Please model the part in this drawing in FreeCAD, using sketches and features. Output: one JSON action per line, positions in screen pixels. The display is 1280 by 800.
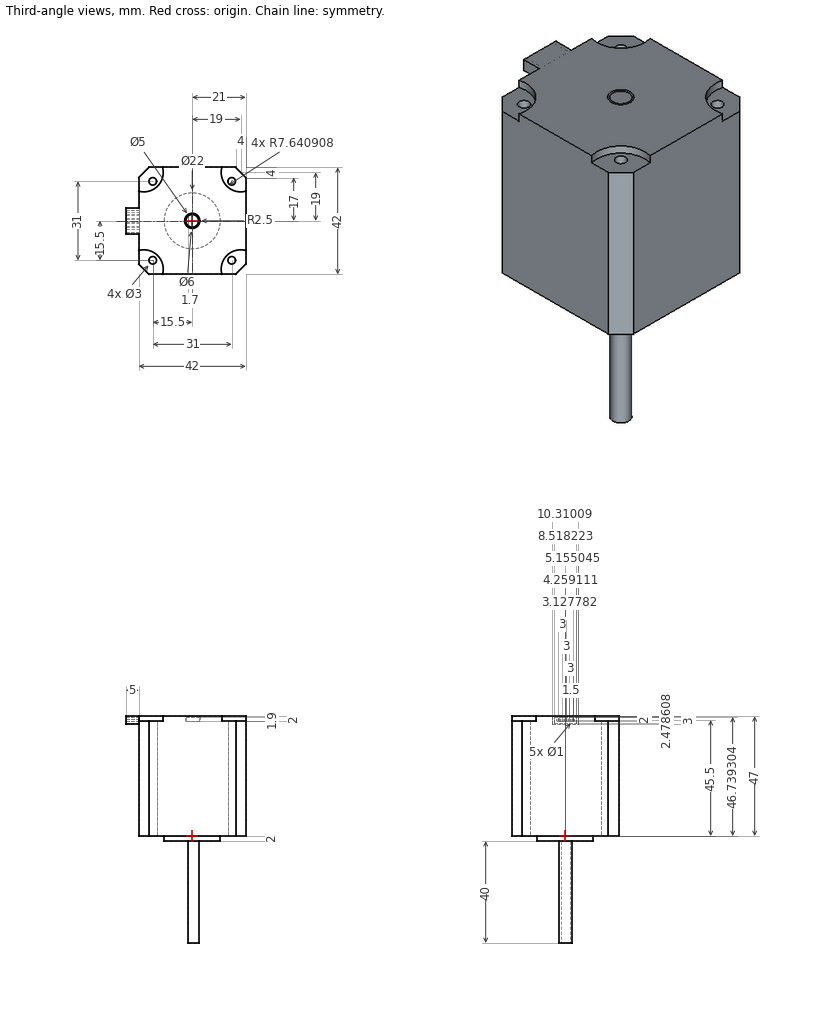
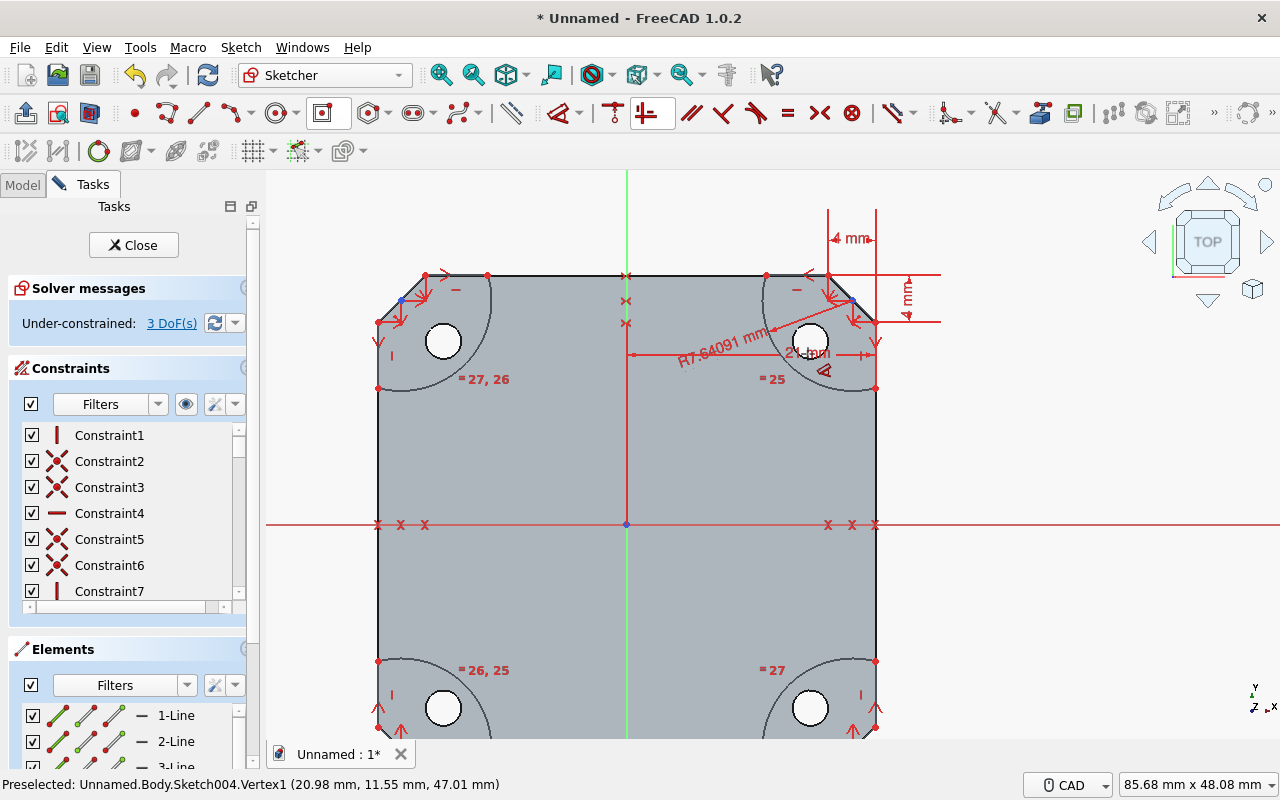
{"action": "left_click", "coordinate": [876, 322]}
{"action": "left_click", "coordinate": [910, 424]}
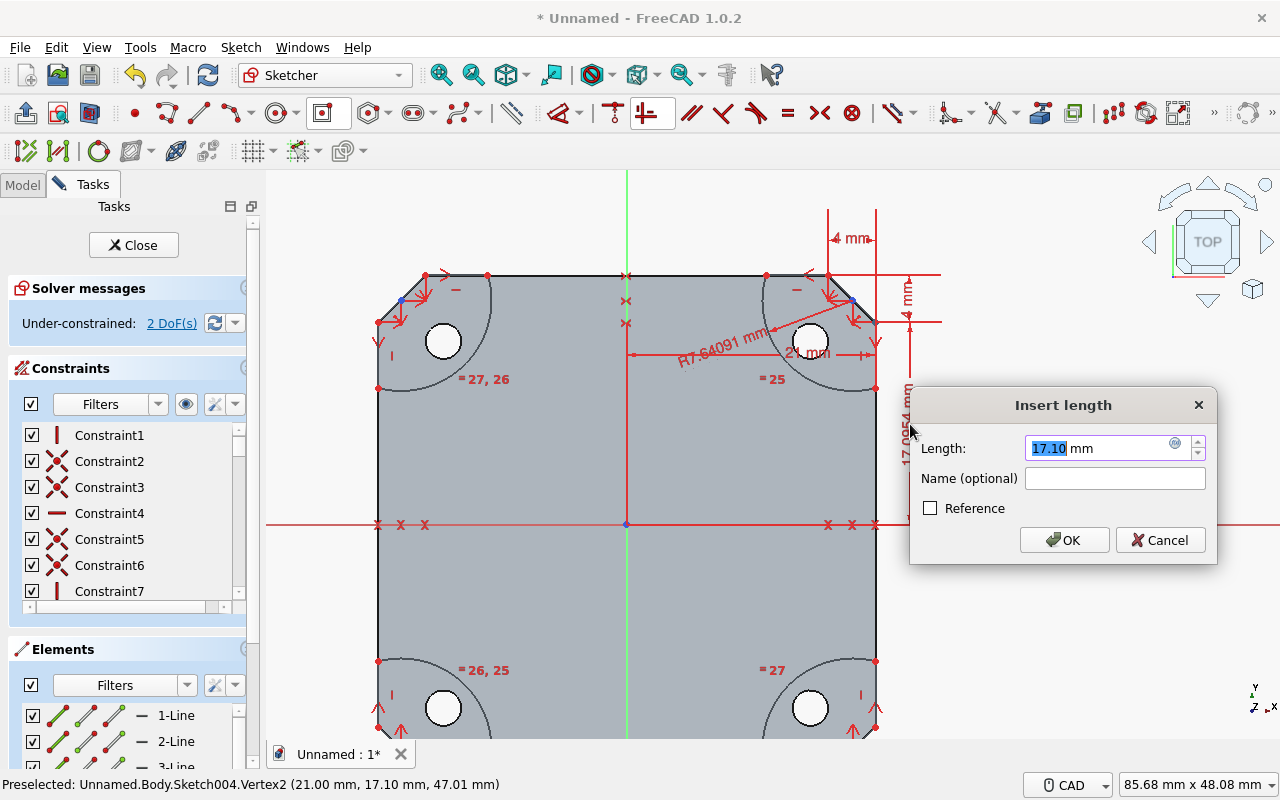
{"action": "type", "text": "17"}
{"action": "key", "text": "Return"}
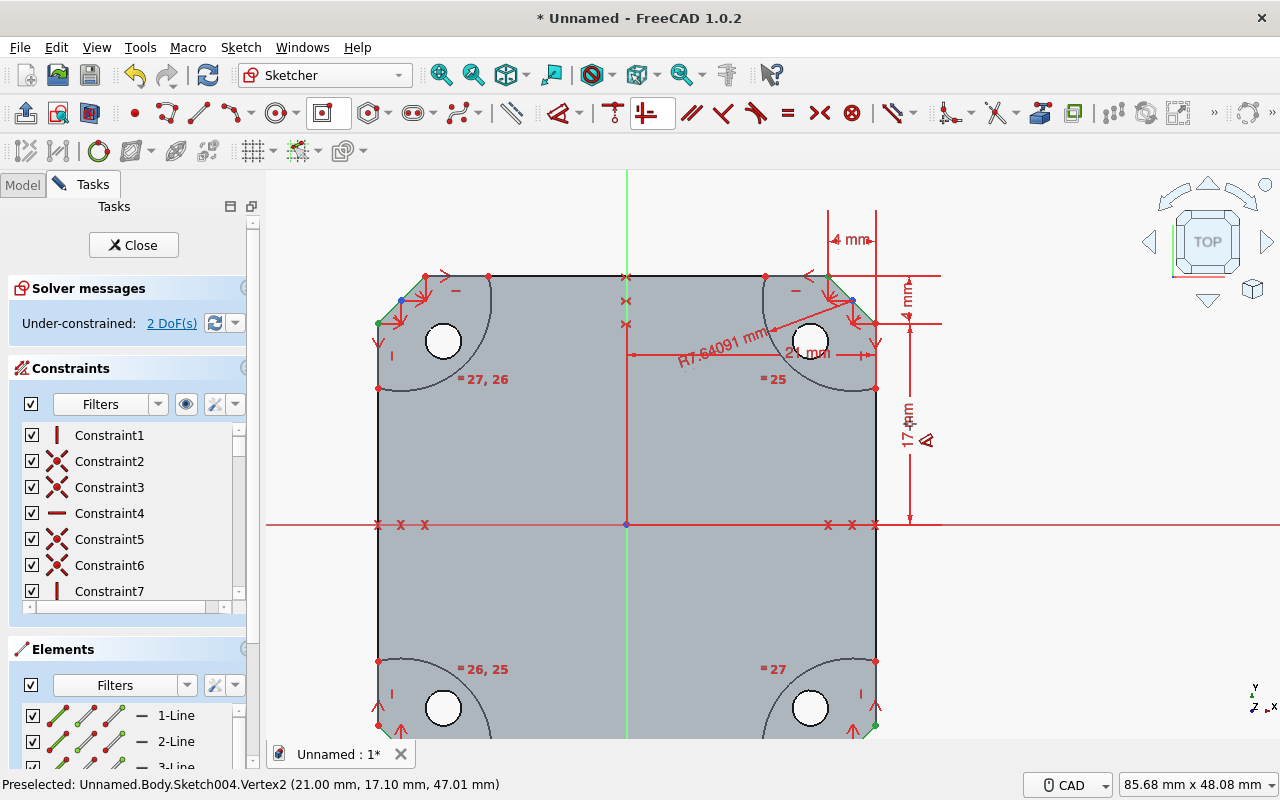
{"action": "left_click", "coordinate": [853, 301]}
{"action": "left_click", "coordinate": [740, 267]}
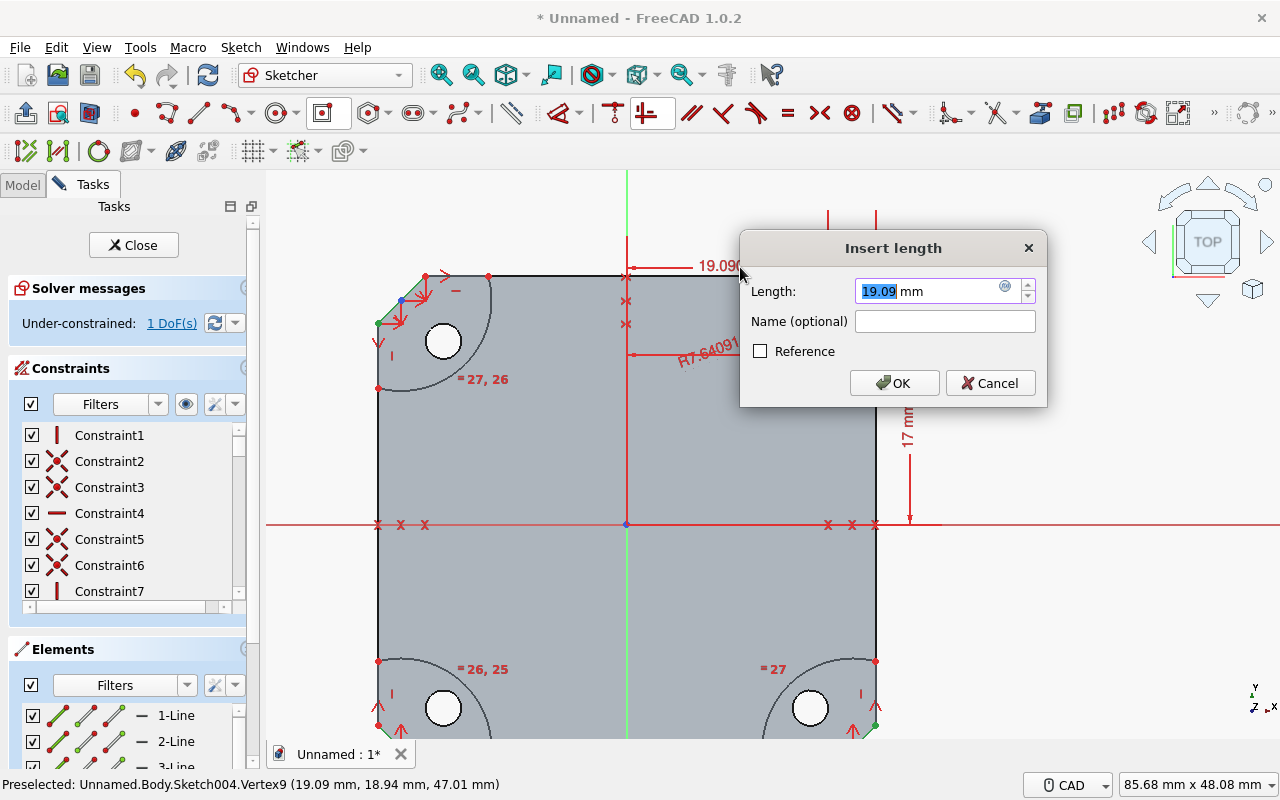
{"action": "type", "text": "19"}
{"action": "key", "text": "Return"}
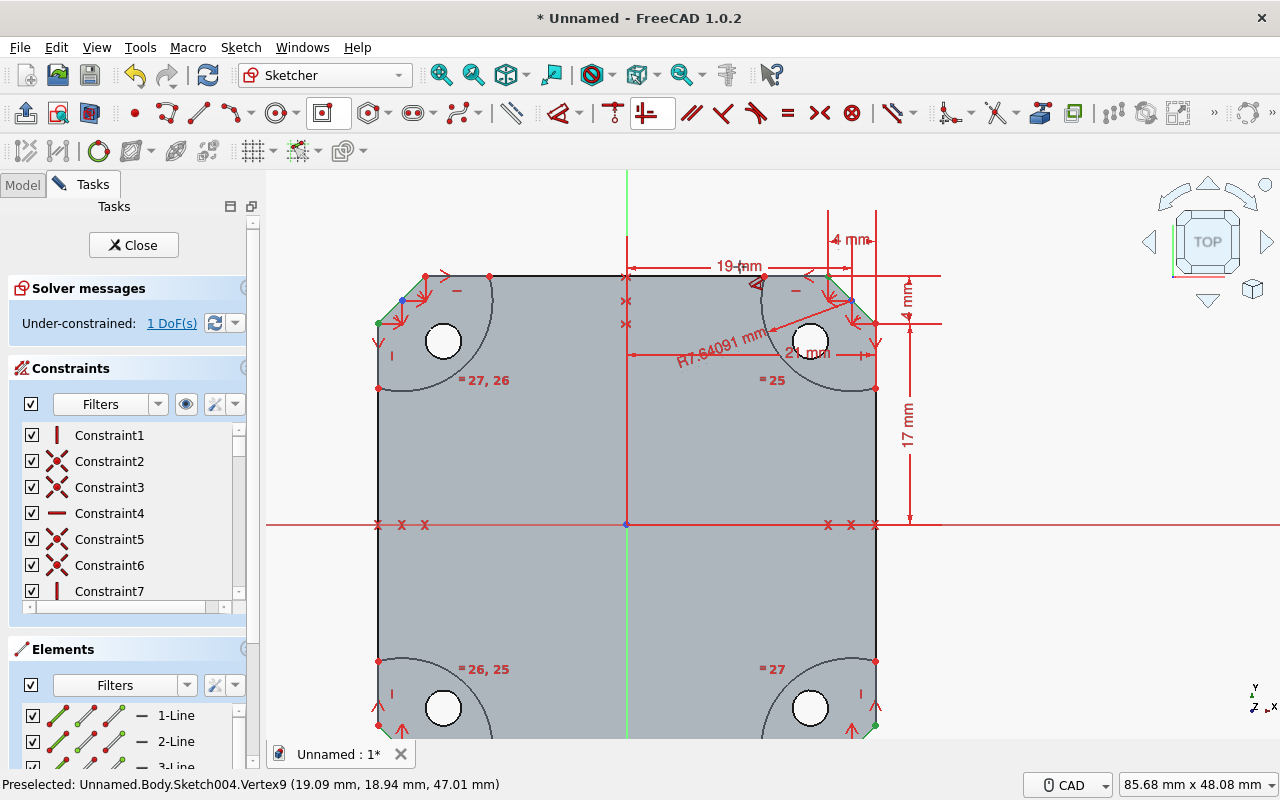
{"action": "left_click", "coordinate": [852, 301]}
{"action": "left_click", "coordinate": [886, 464]}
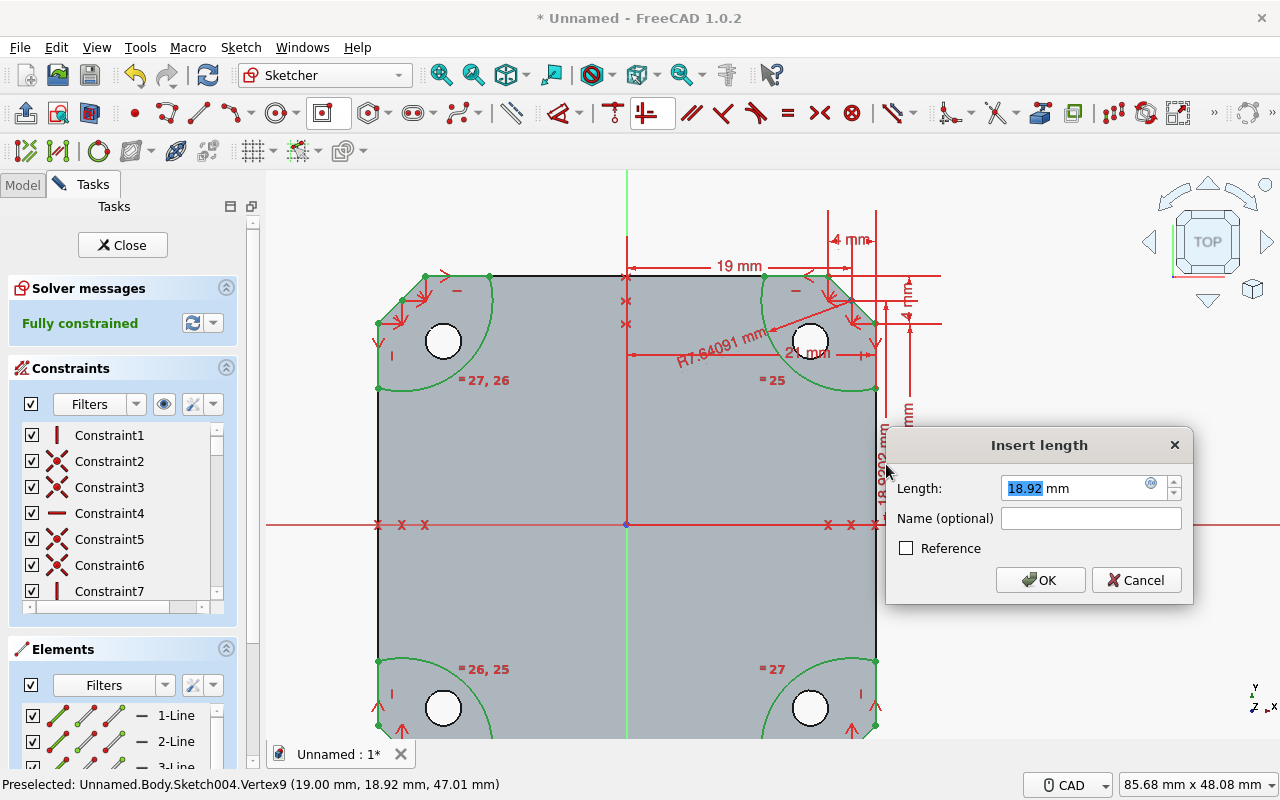
{"action": "type", "text": "19"}
{"action": "key", "text": "Return"}
{"action": "key", "text": "Escape"}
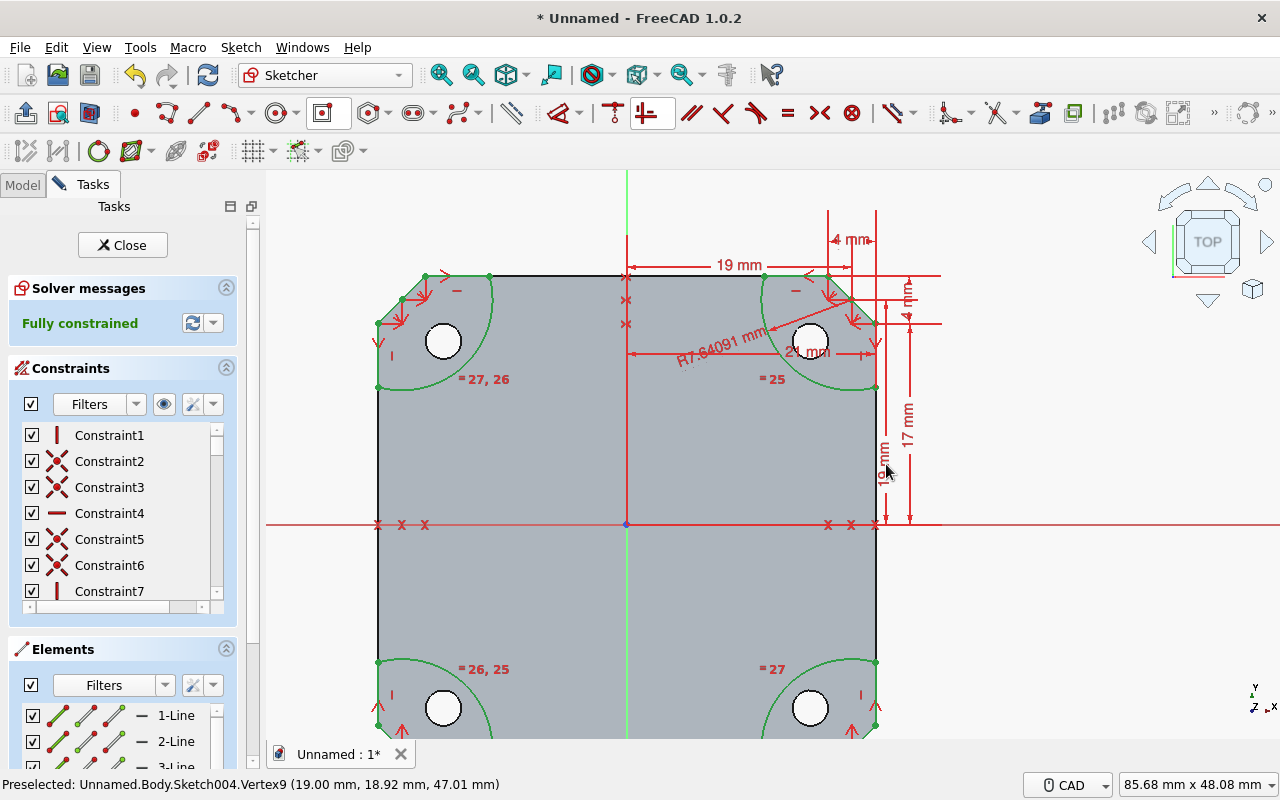
{"action": "left_click", "coordinate": [123, 245]}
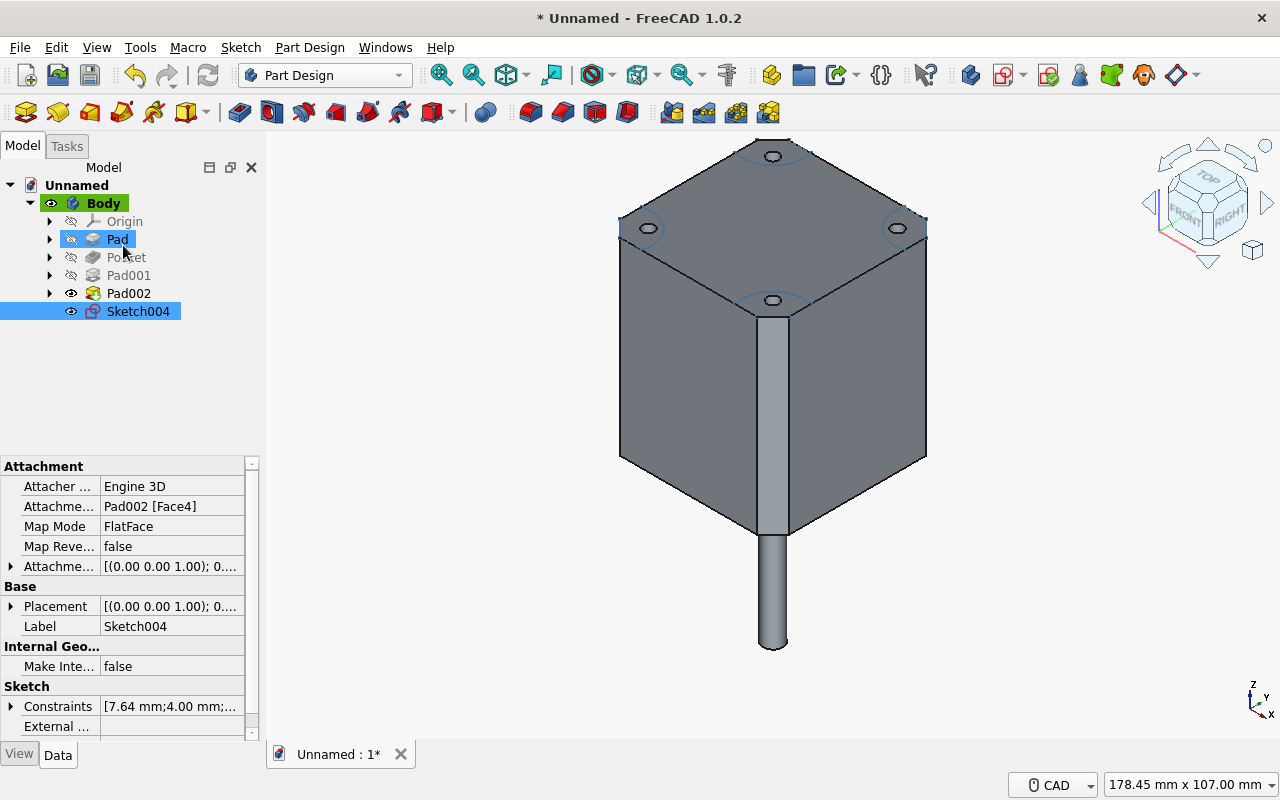
{"action": "left_click", "coordinate": [240, 112]}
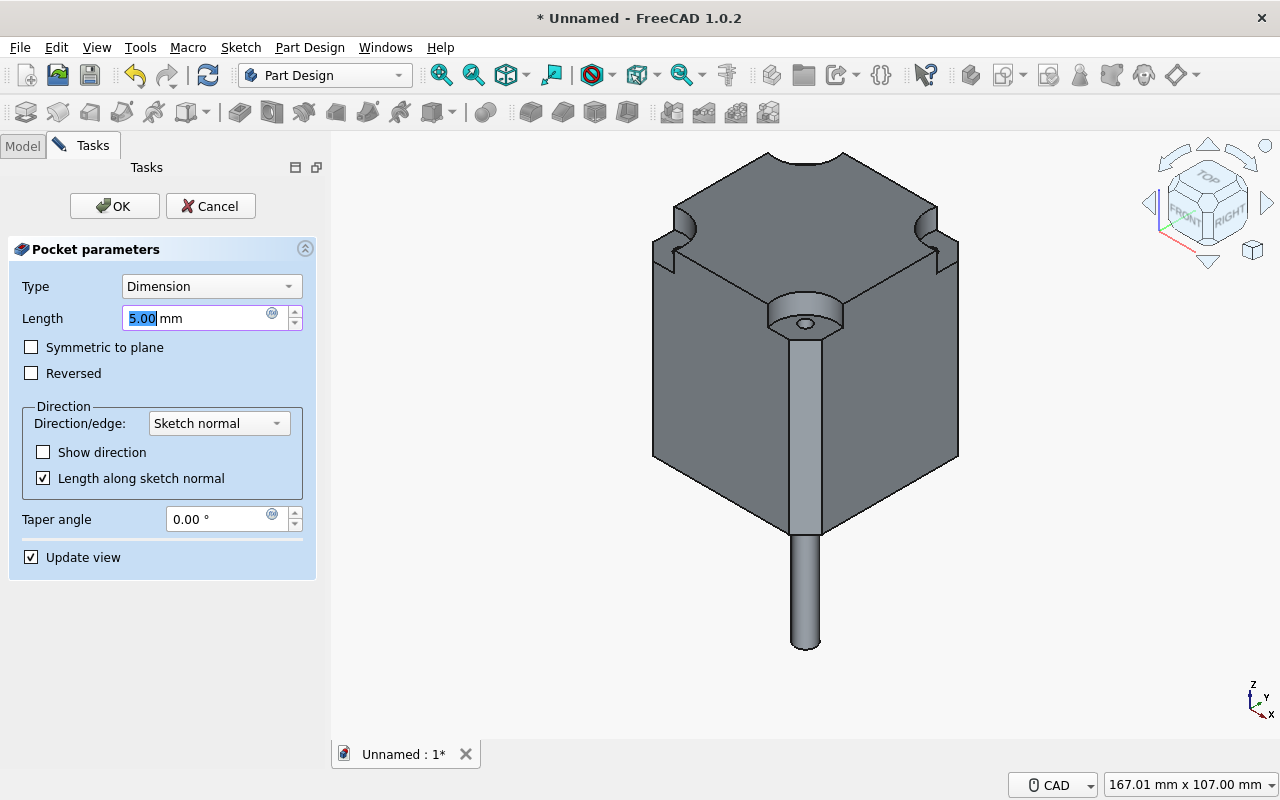
{"action": "type", "text": "2"}
{"action": "key", "text": "Tab"}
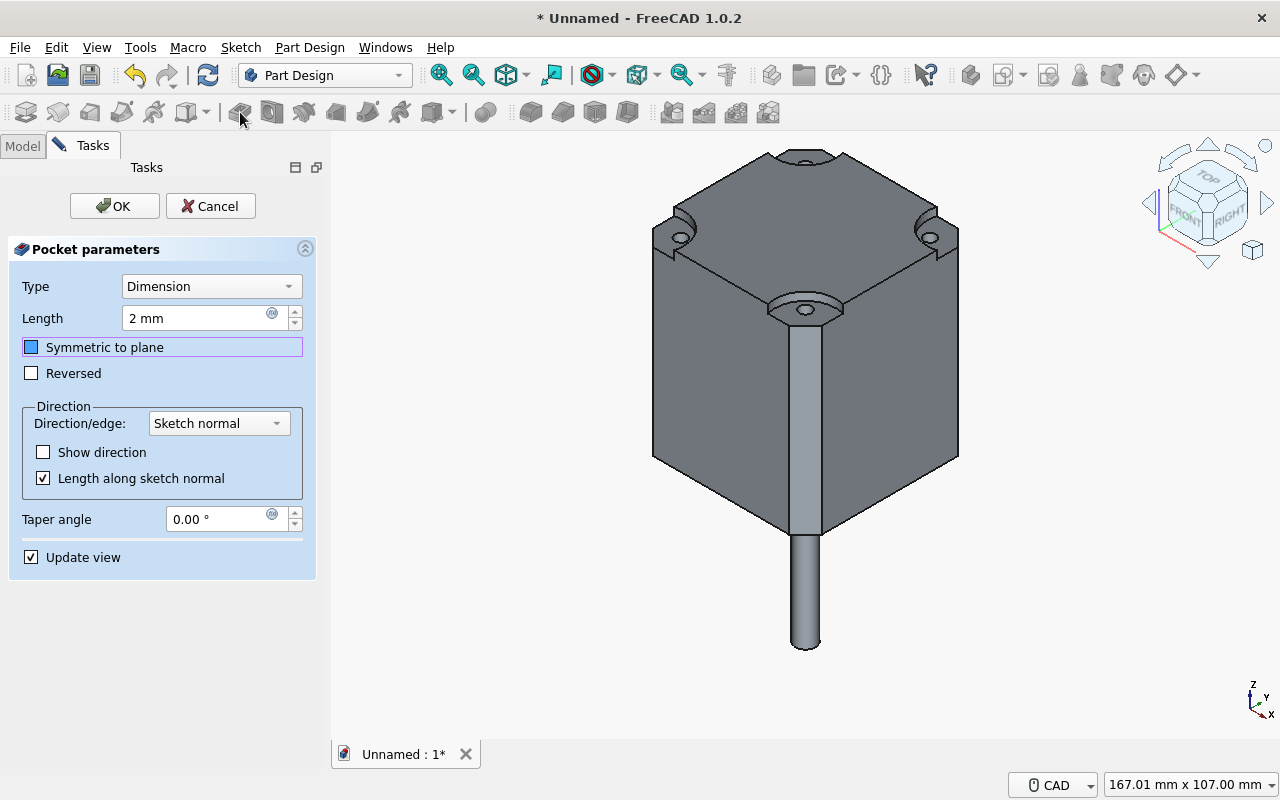
{"action": "left_click", "coordinate": [115, 206]}